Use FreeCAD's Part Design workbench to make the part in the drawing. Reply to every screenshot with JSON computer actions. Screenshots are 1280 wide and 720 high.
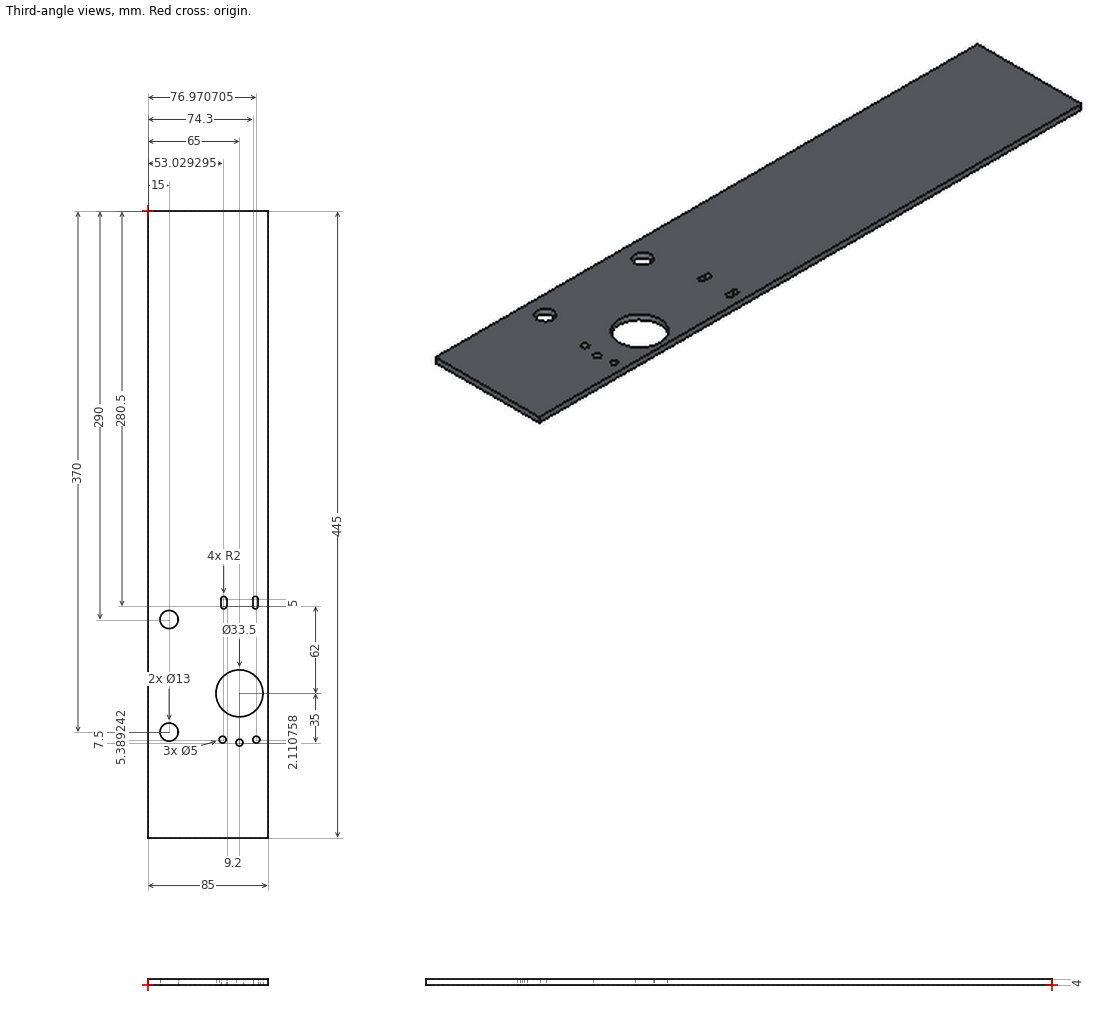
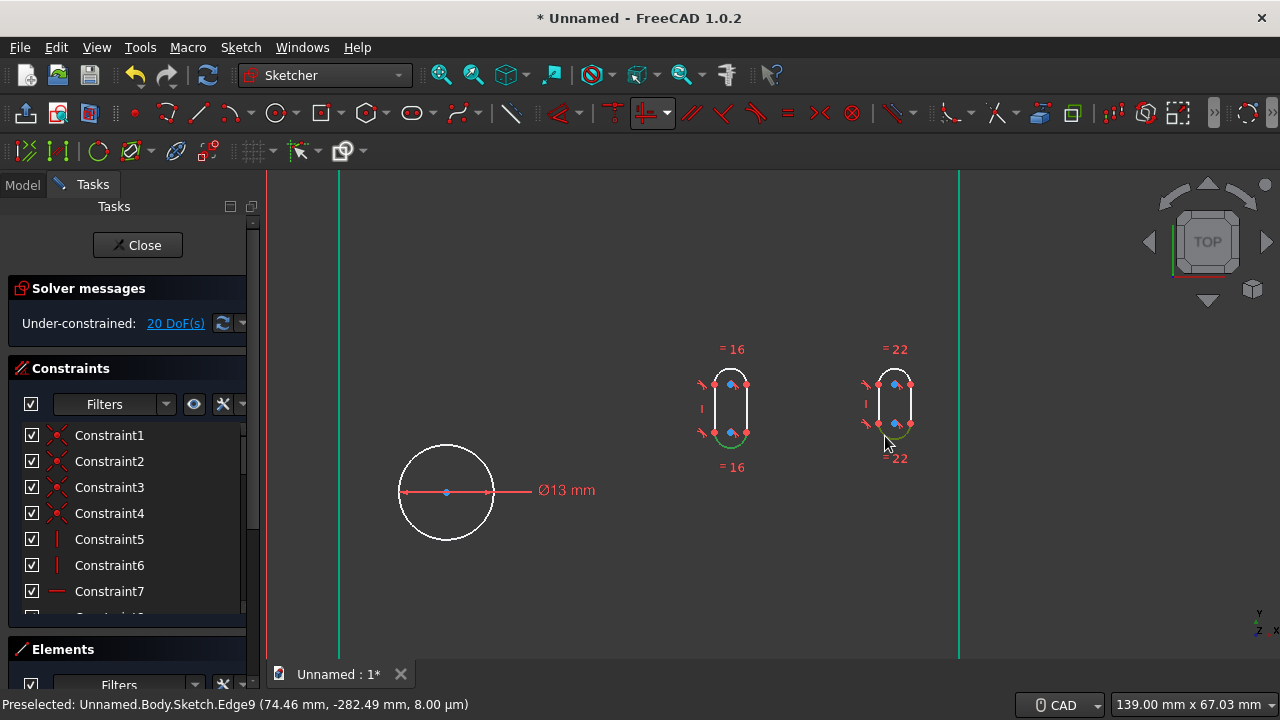
{"action": "left_click", "coordinate": [788, 114]}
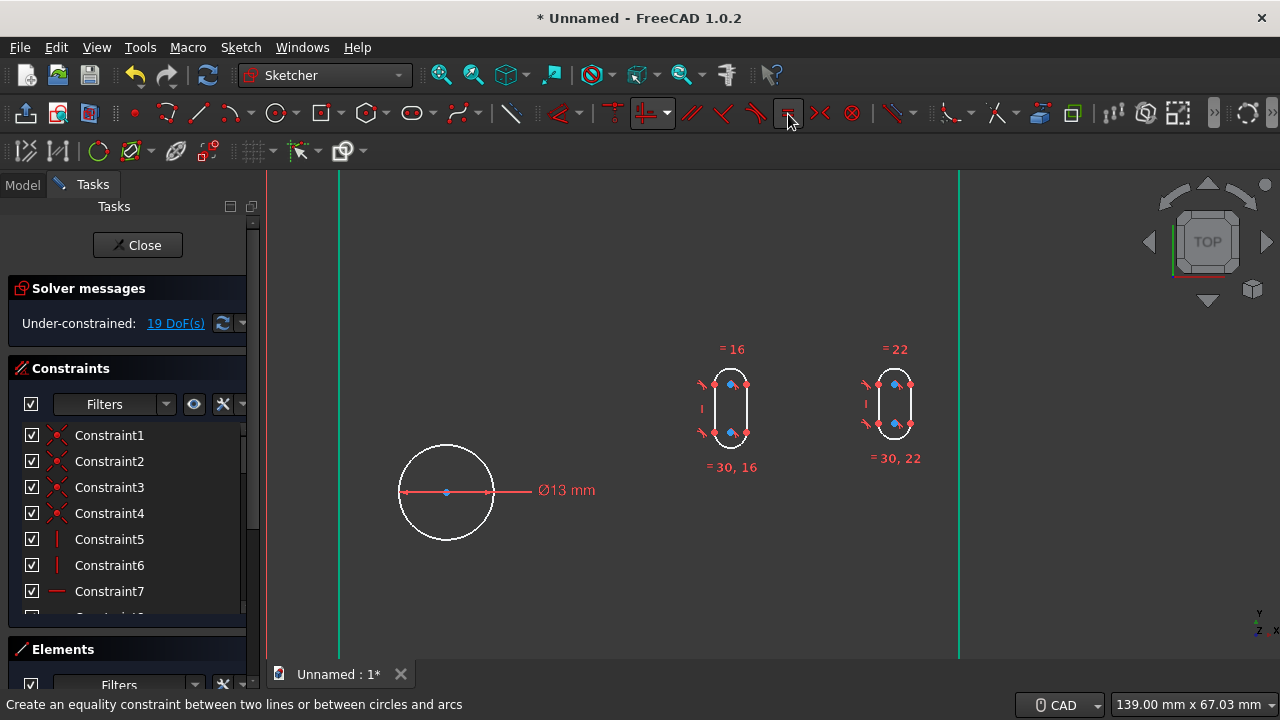
{"action": "key", "text": "d"}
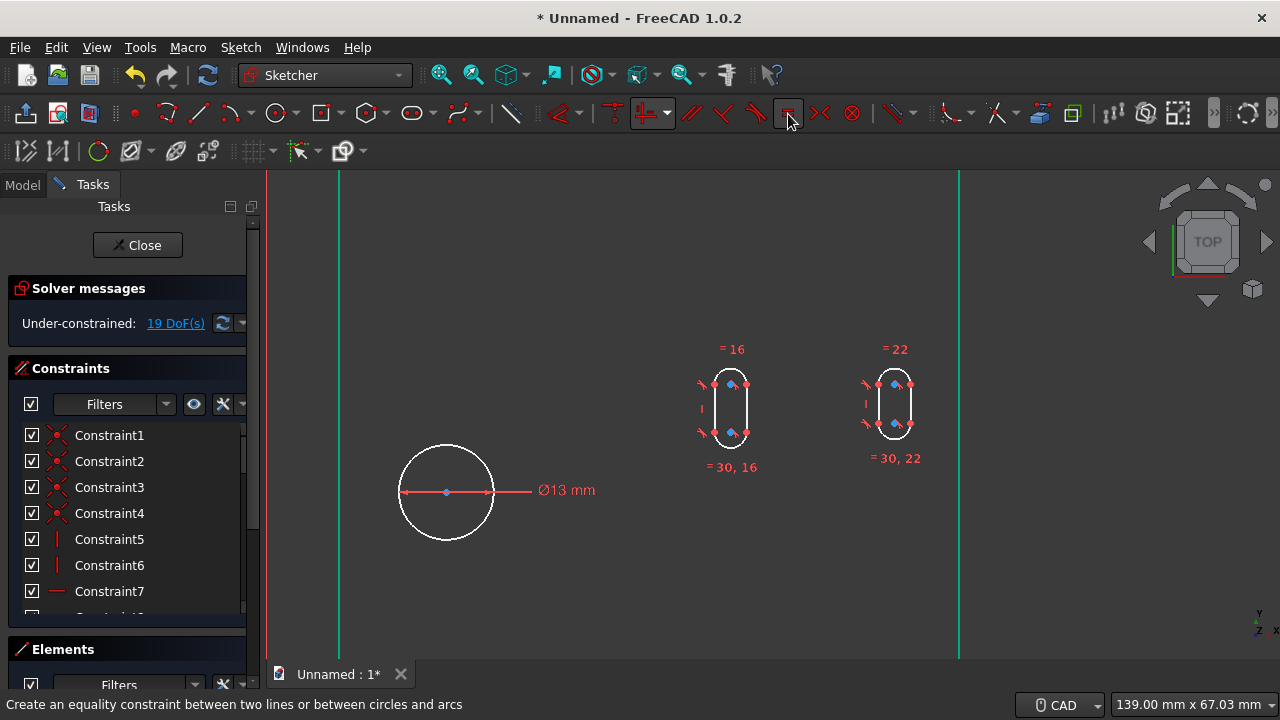
{"action": "scroll", "coordinate": [721, 445], "scroll_direction": "up", "scroll_amount": 6}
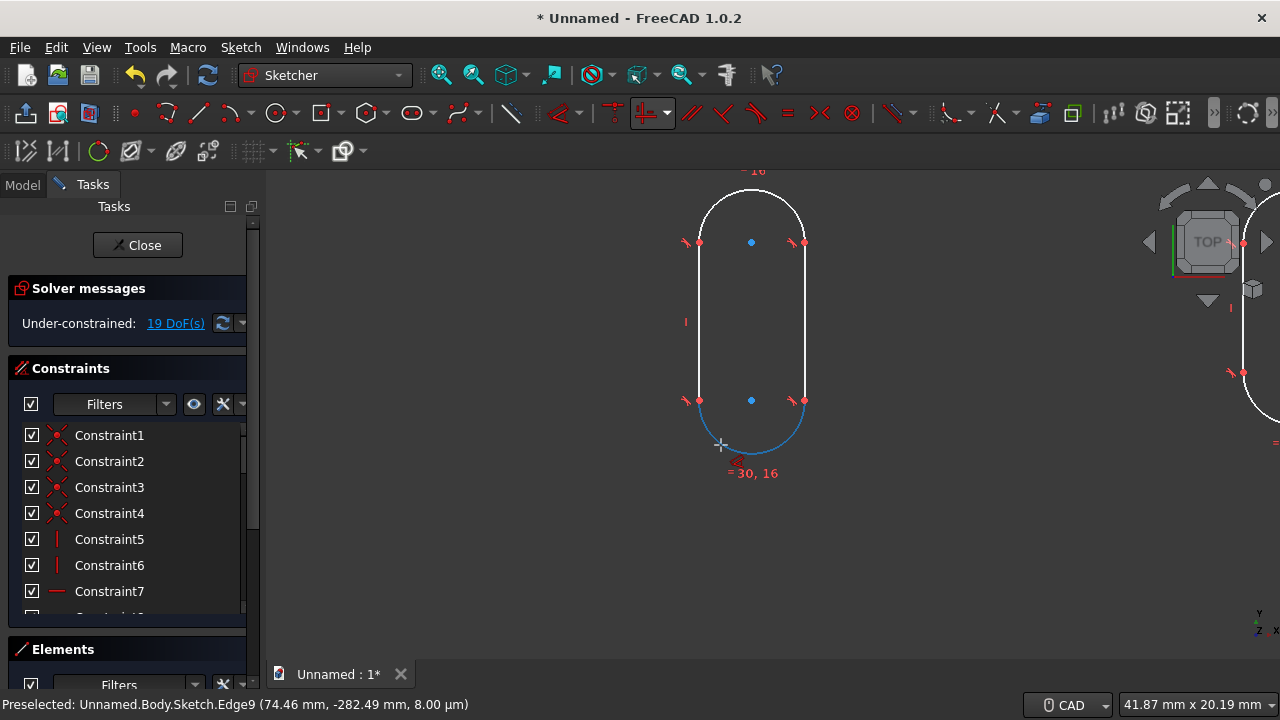
{"action": "left_click", "coordinate": [721, 444]}
{"action": "left_click", "coordinate": [702, 470]}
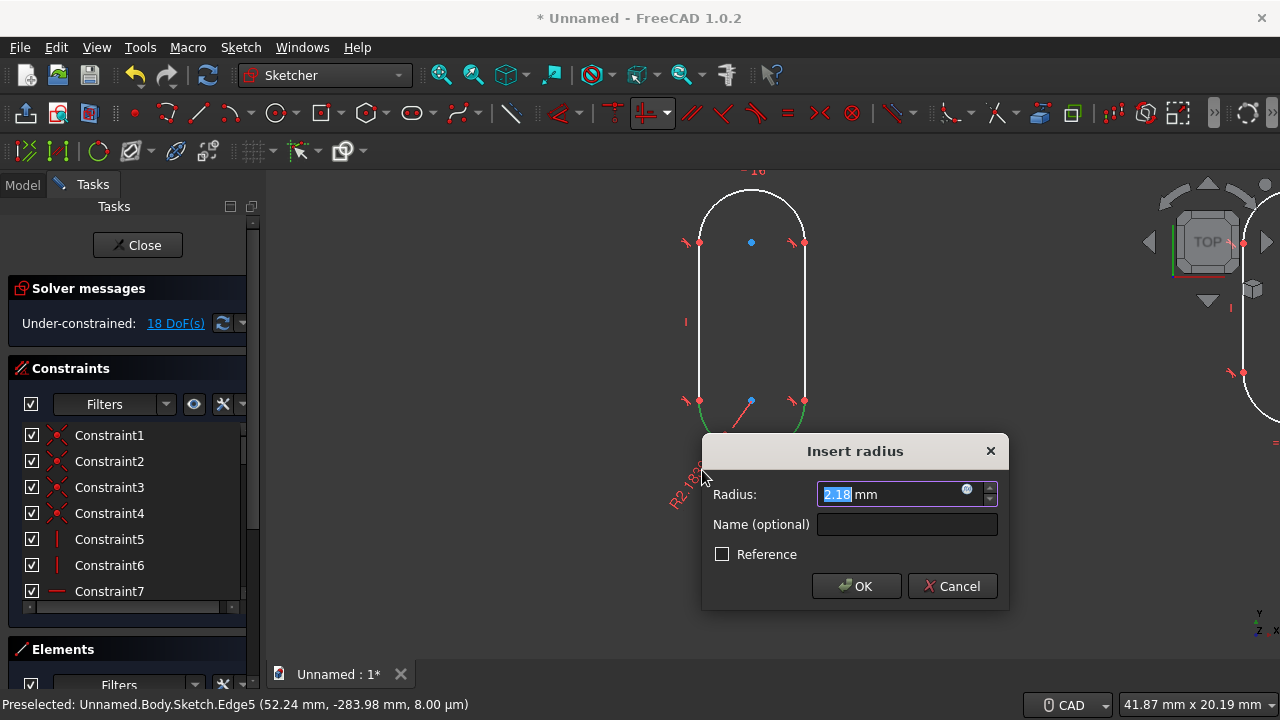
{"action": "type", "text": "2"}
{"action": "key", "text": "Return"}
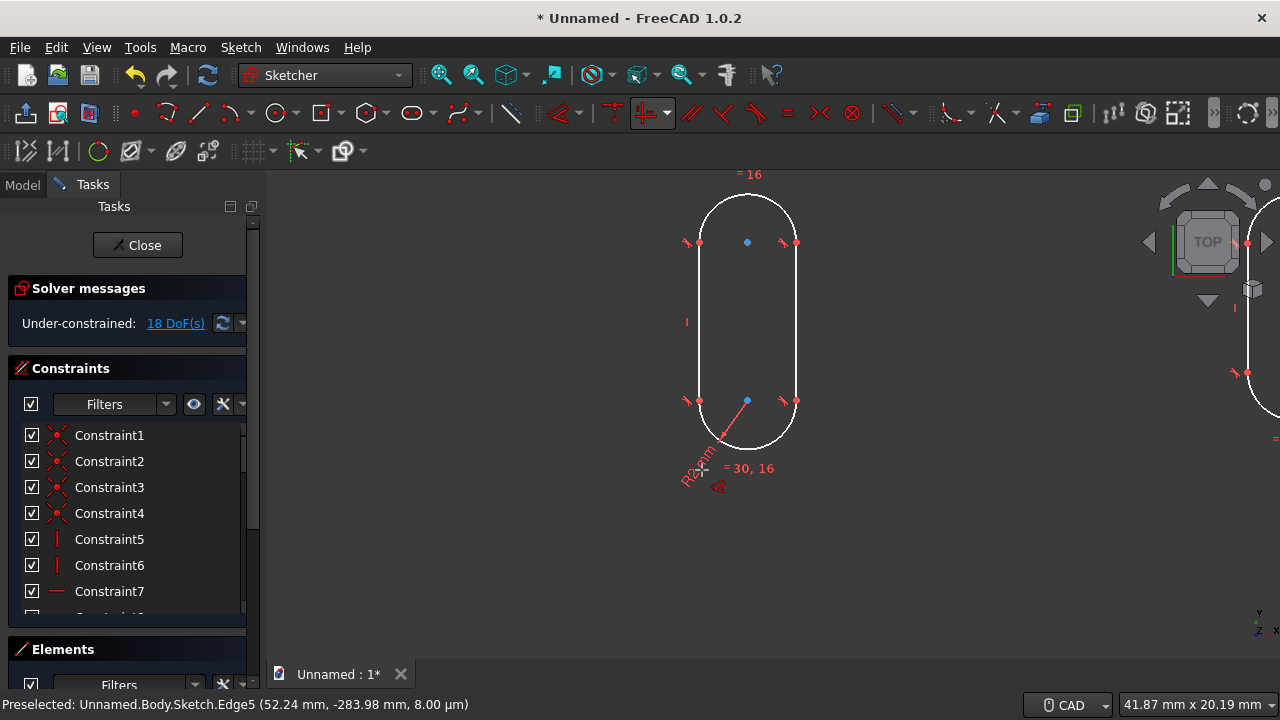
{"action": "scroll", "coordinate": [712, 465], "scroll_direction": "down", "scroll_amount": 17}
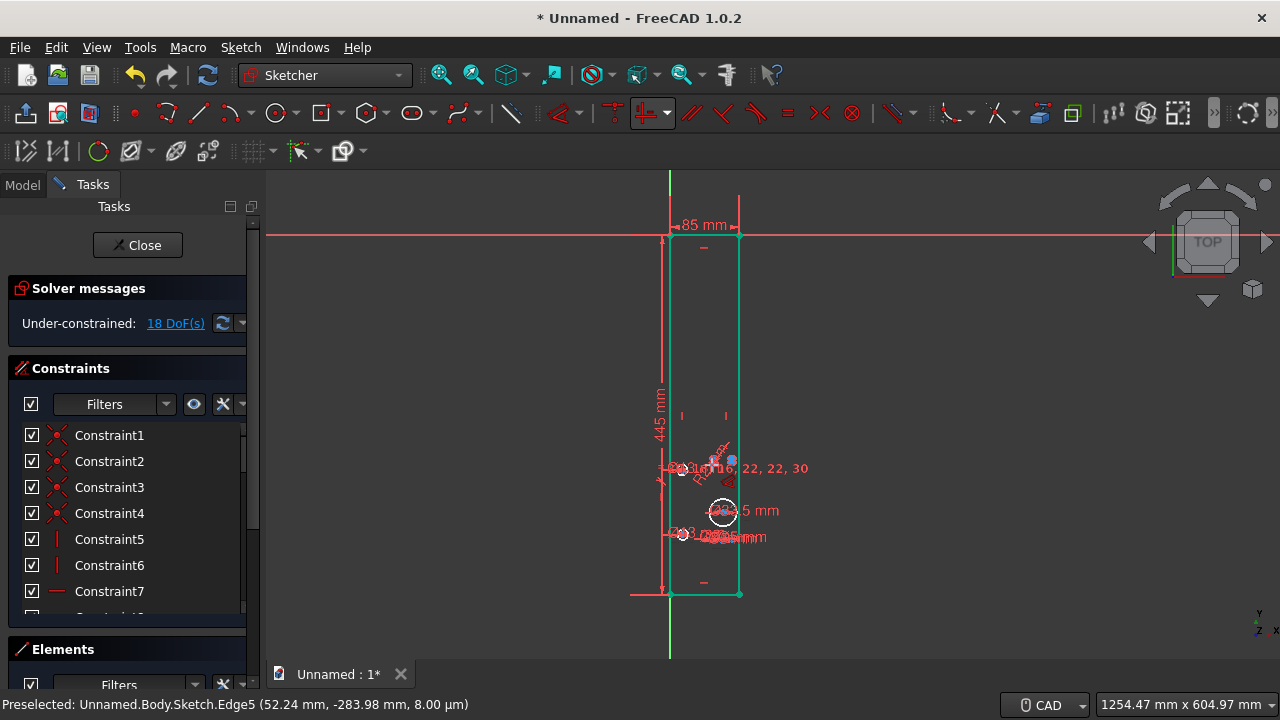
{"action": "scroll", "coordinate": [712, 462], "scroll_direction": "up", "scroll_amount": 12}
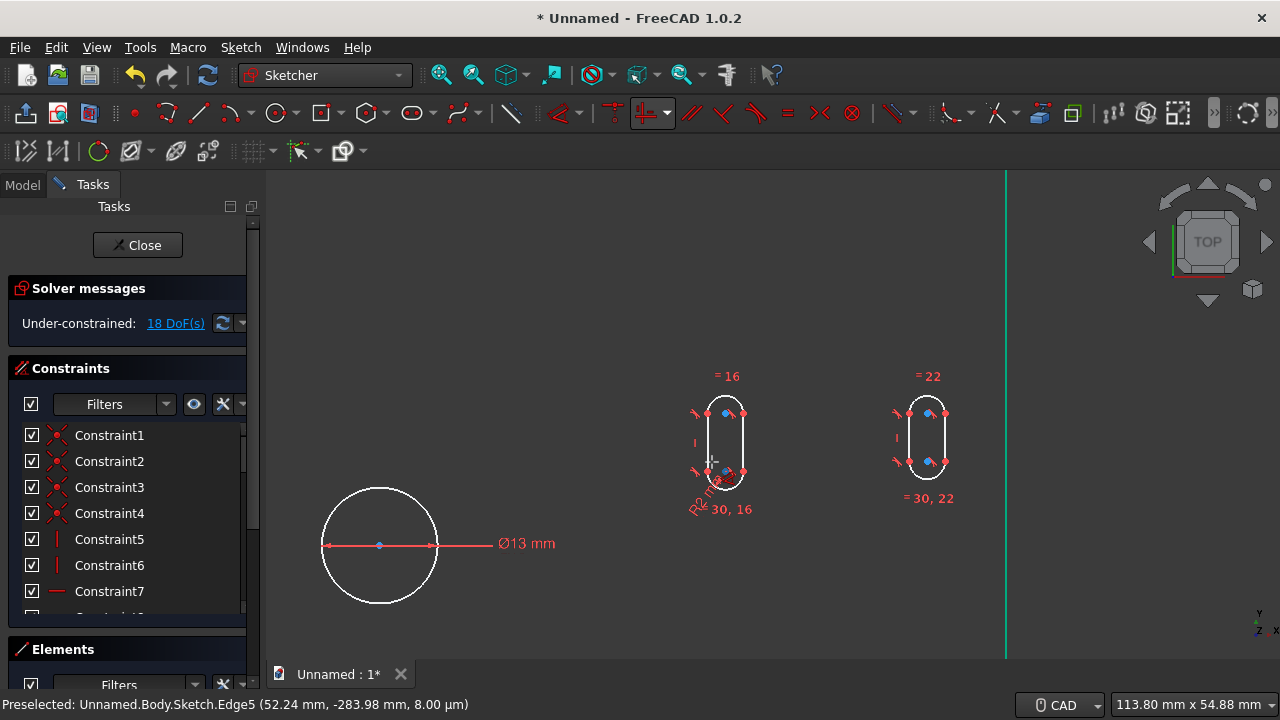
{"action": "left_click", "coordinate": [708, 454]}
{"action": "left_click", "coordinate": [674, 443]}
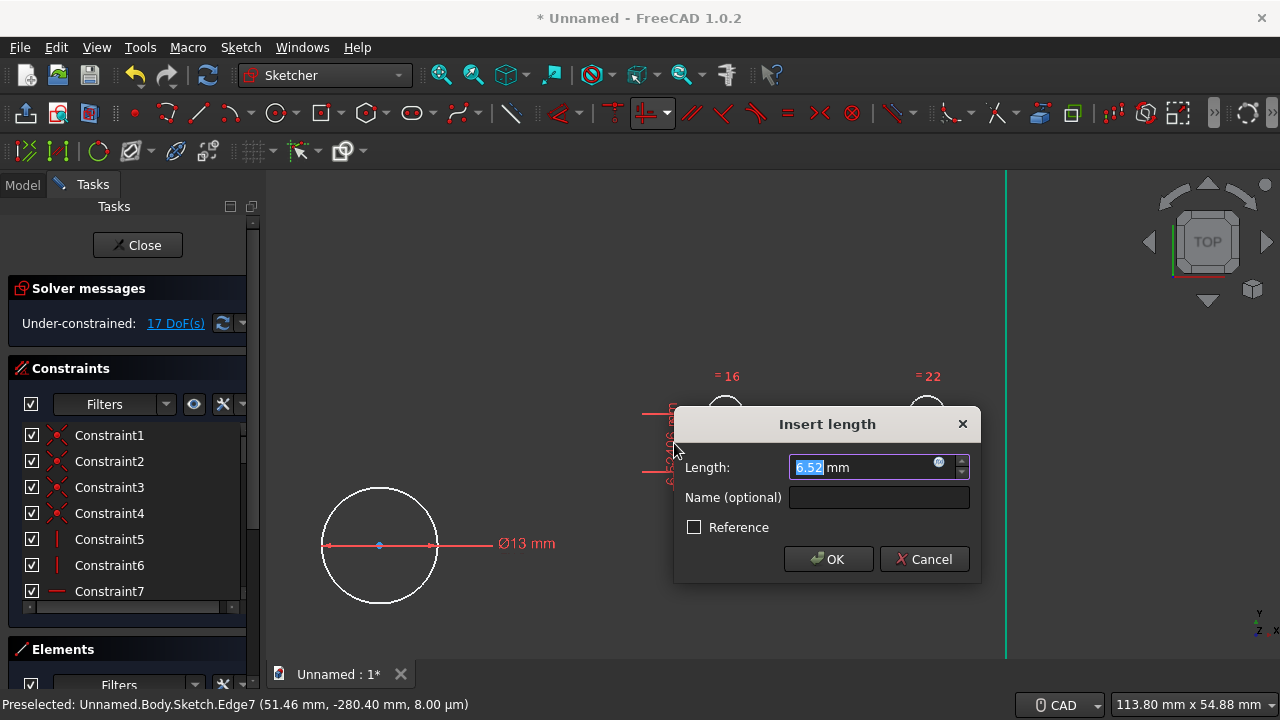
{"action": "type", "text": "5"}
{"action": "key", "text": "Return"}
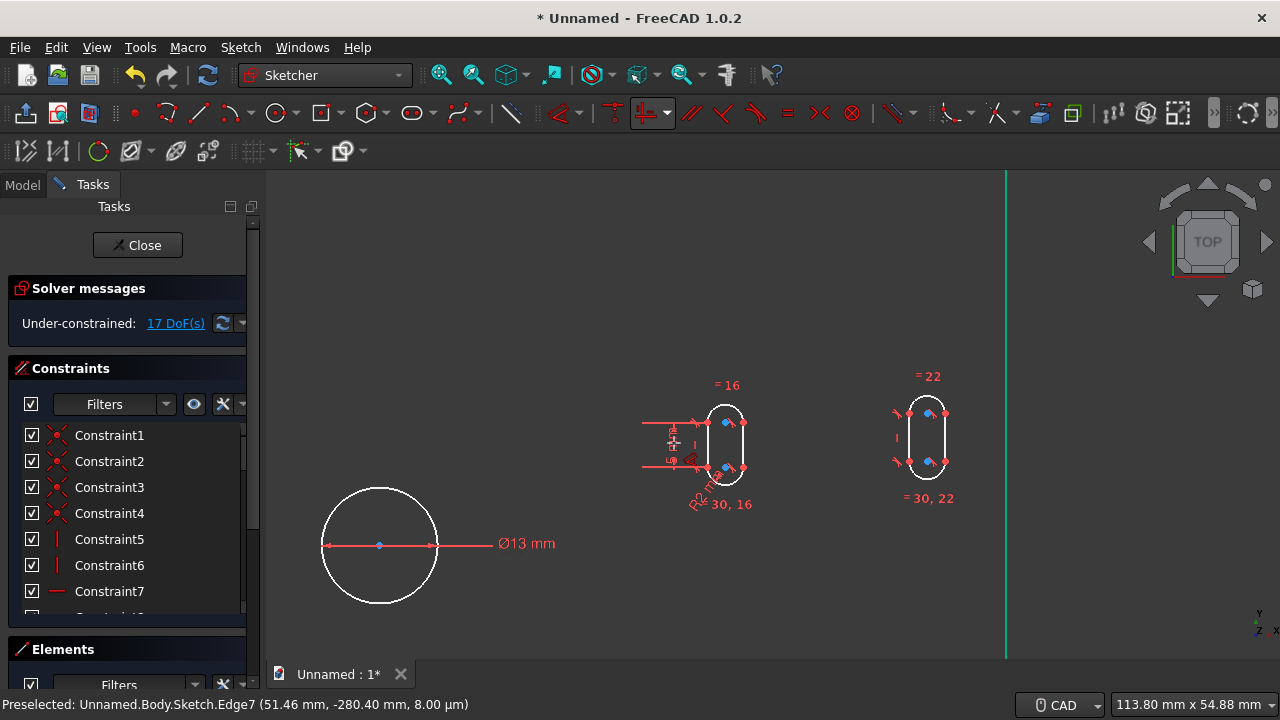
{"action": "left_click", "coordinate": [909, 447]}
{"action": "left_click", "coordinate": [875, 438]}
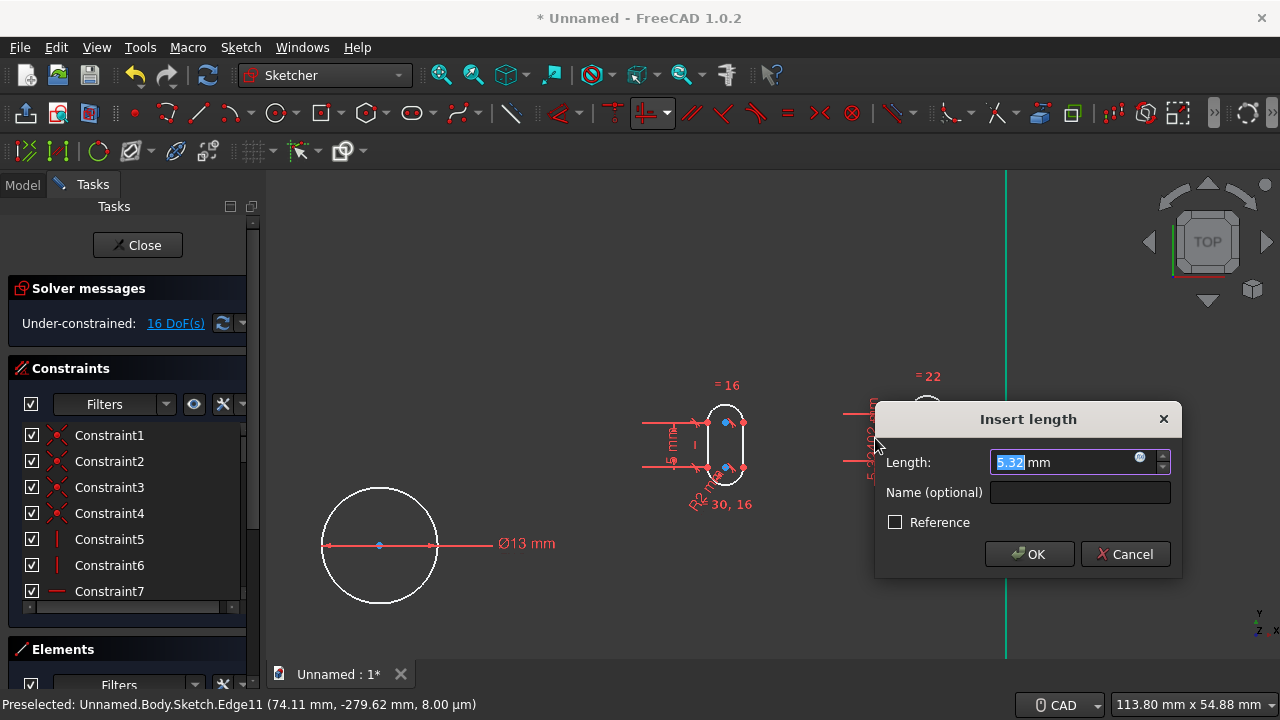
{"action": "type", "text": "5"}
{"action": "key", "text": "Return"}